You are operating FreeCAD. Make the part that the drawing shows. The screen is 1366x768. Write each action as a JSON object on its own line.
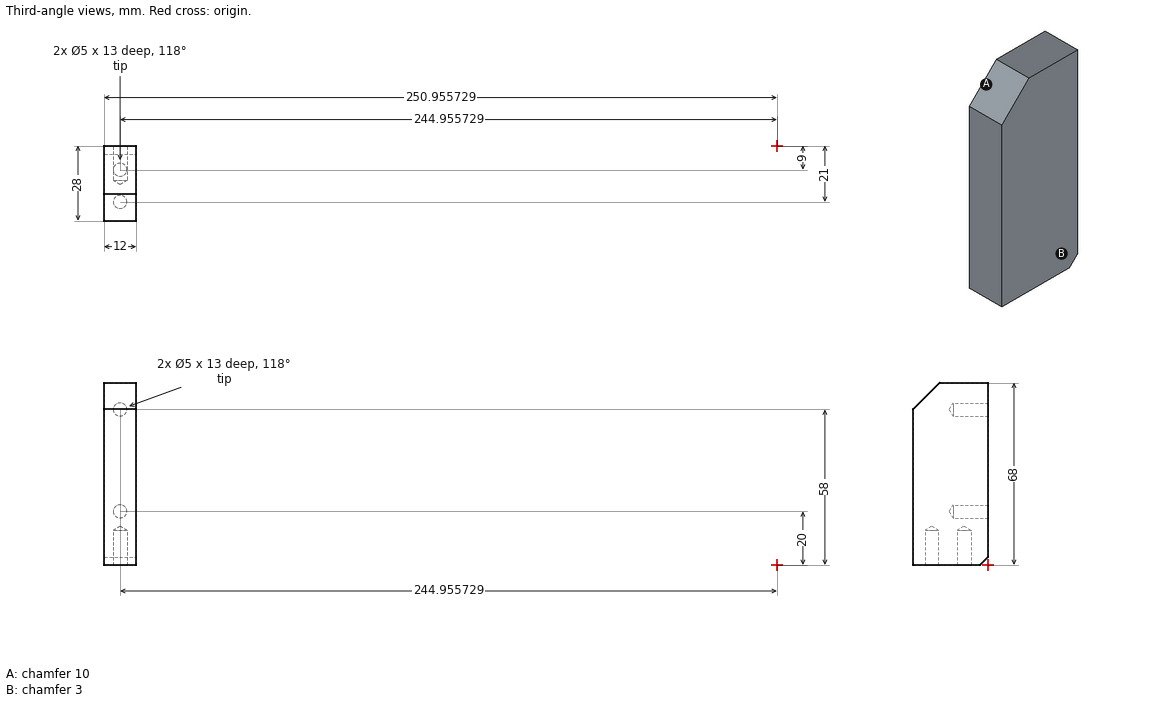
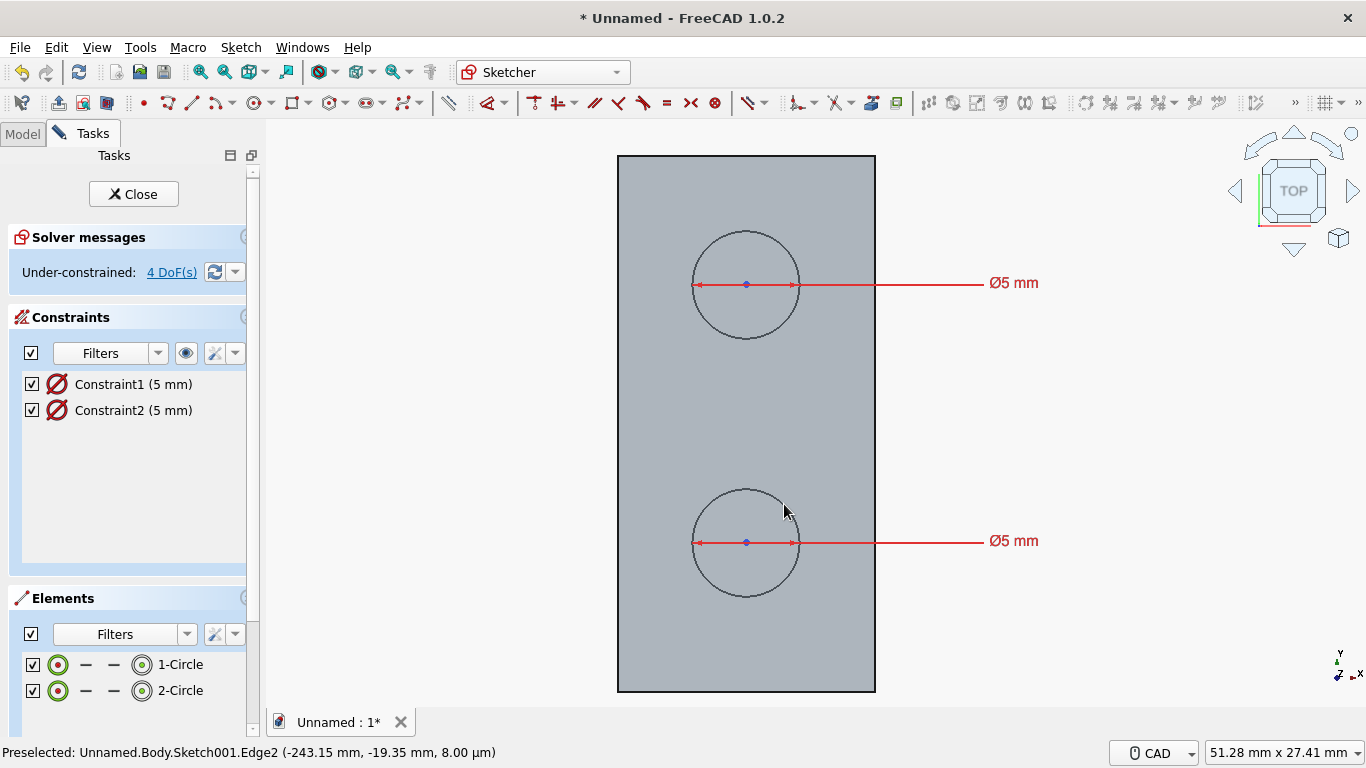
{"action": "left_click", "coordinate": [488, 104]}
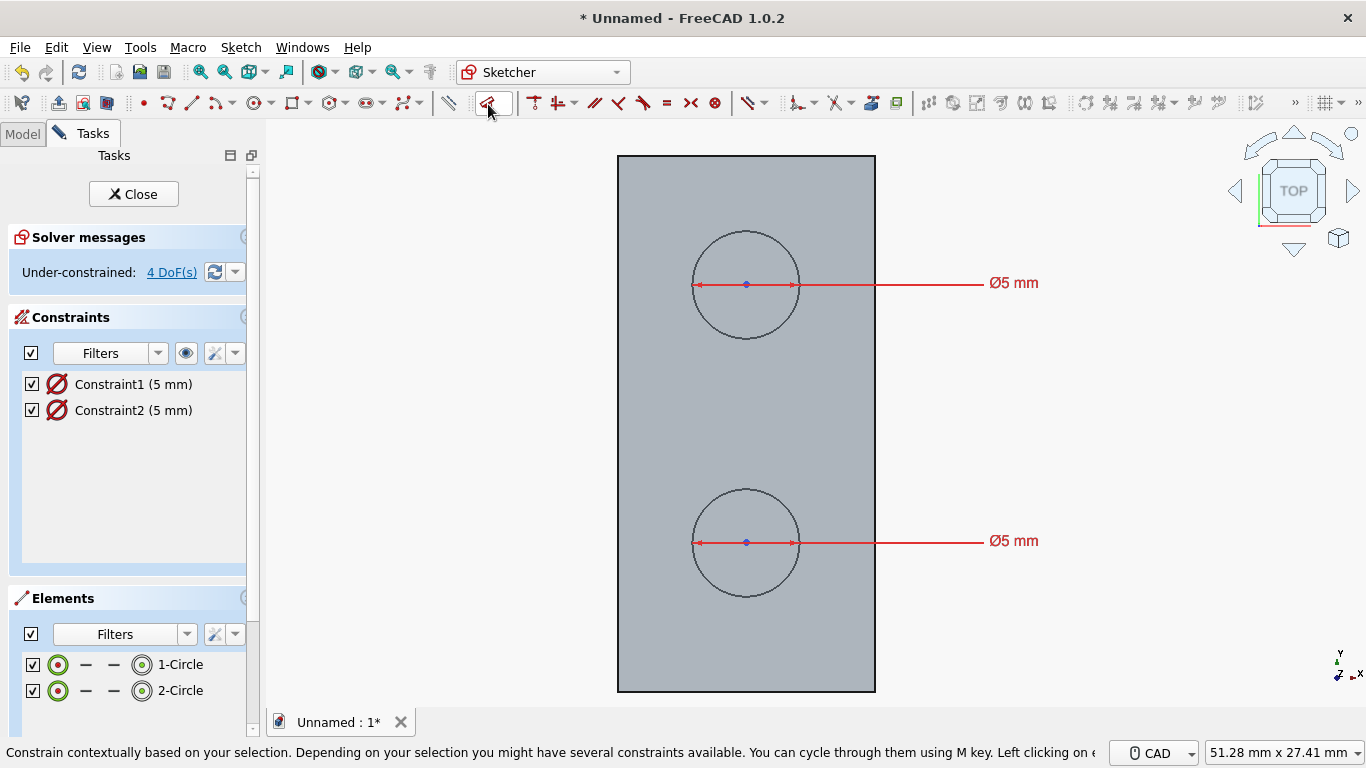
{"action": "left_click", "coordinate": [746, 285]}
{"action": "left_click", "coordinate": [712, 216]}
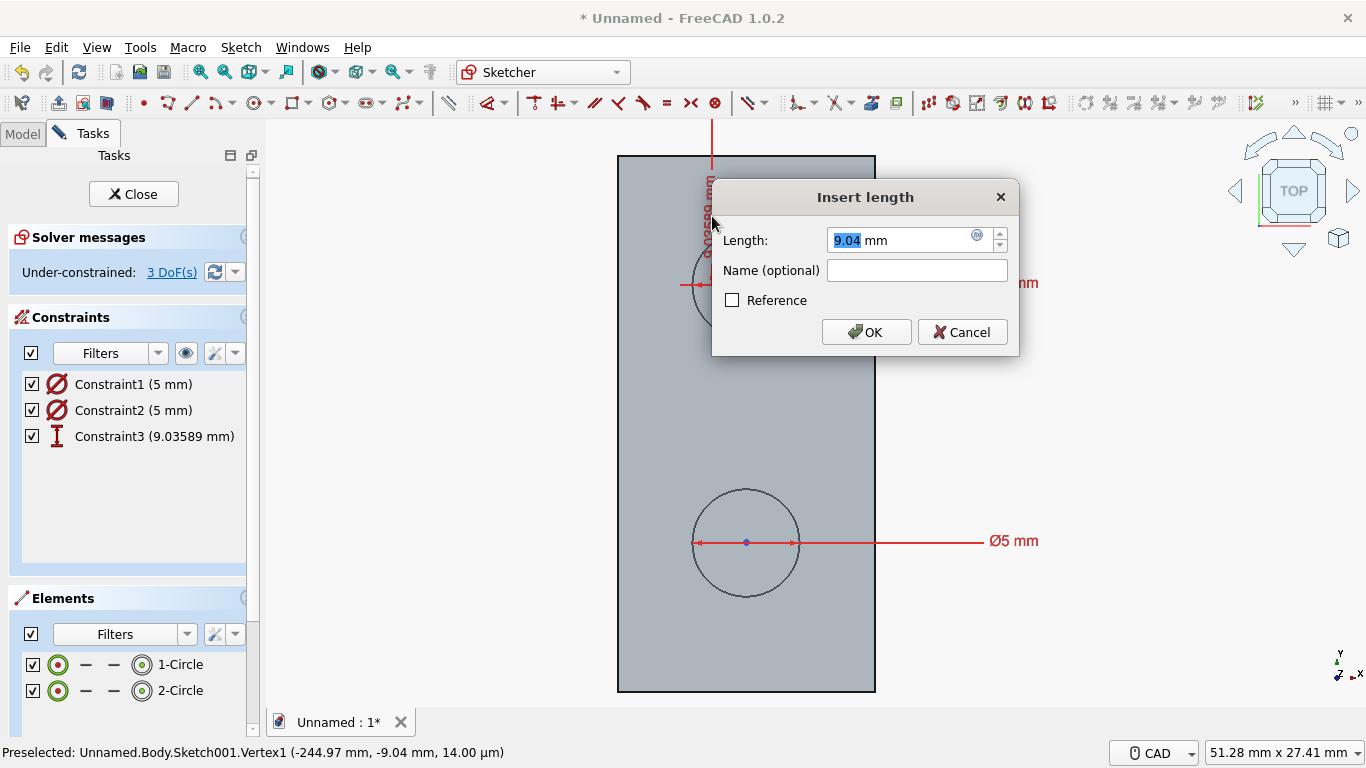
{"action": "type", "text": "9"}
{"action": "key", "text": "Return"}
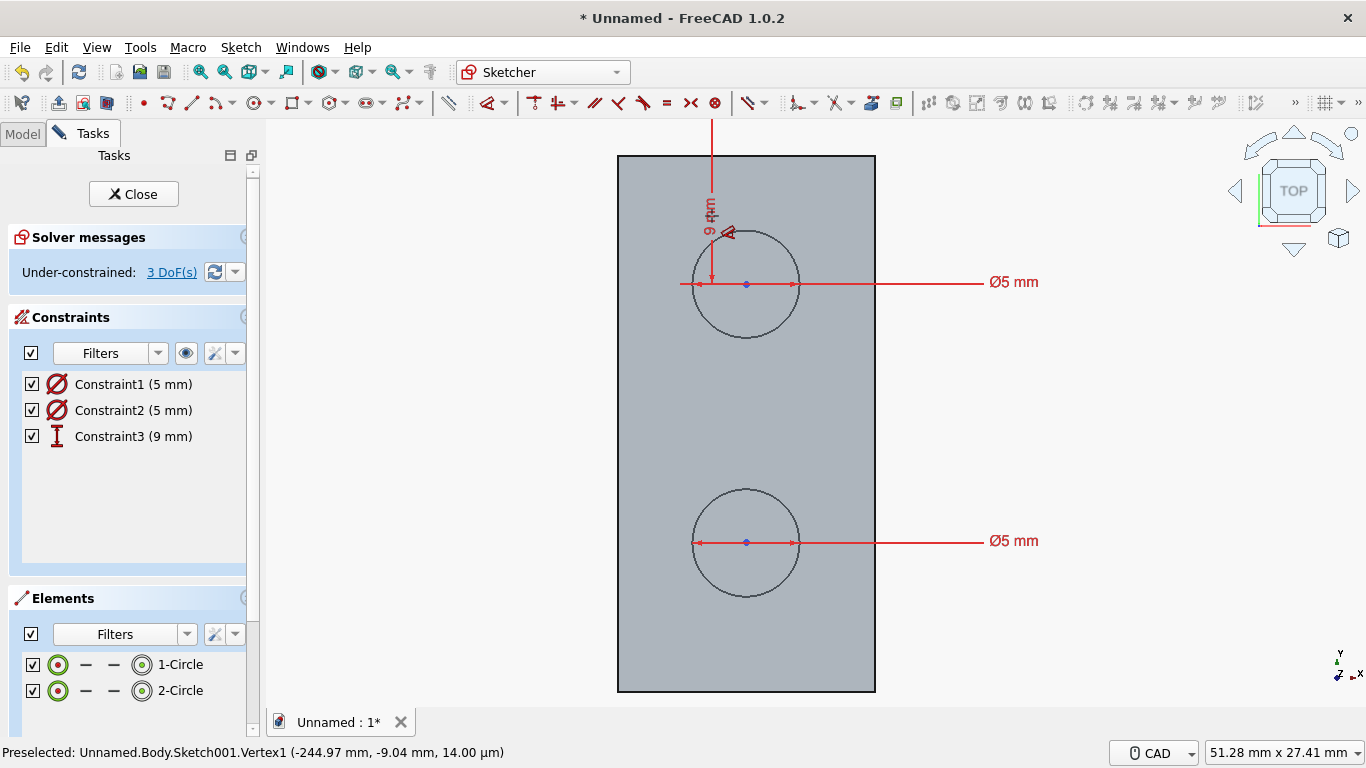
{"action": "left_click", "coordinate": [746, 543]}
{"action": "left_click", "coordinate": [712, 345]}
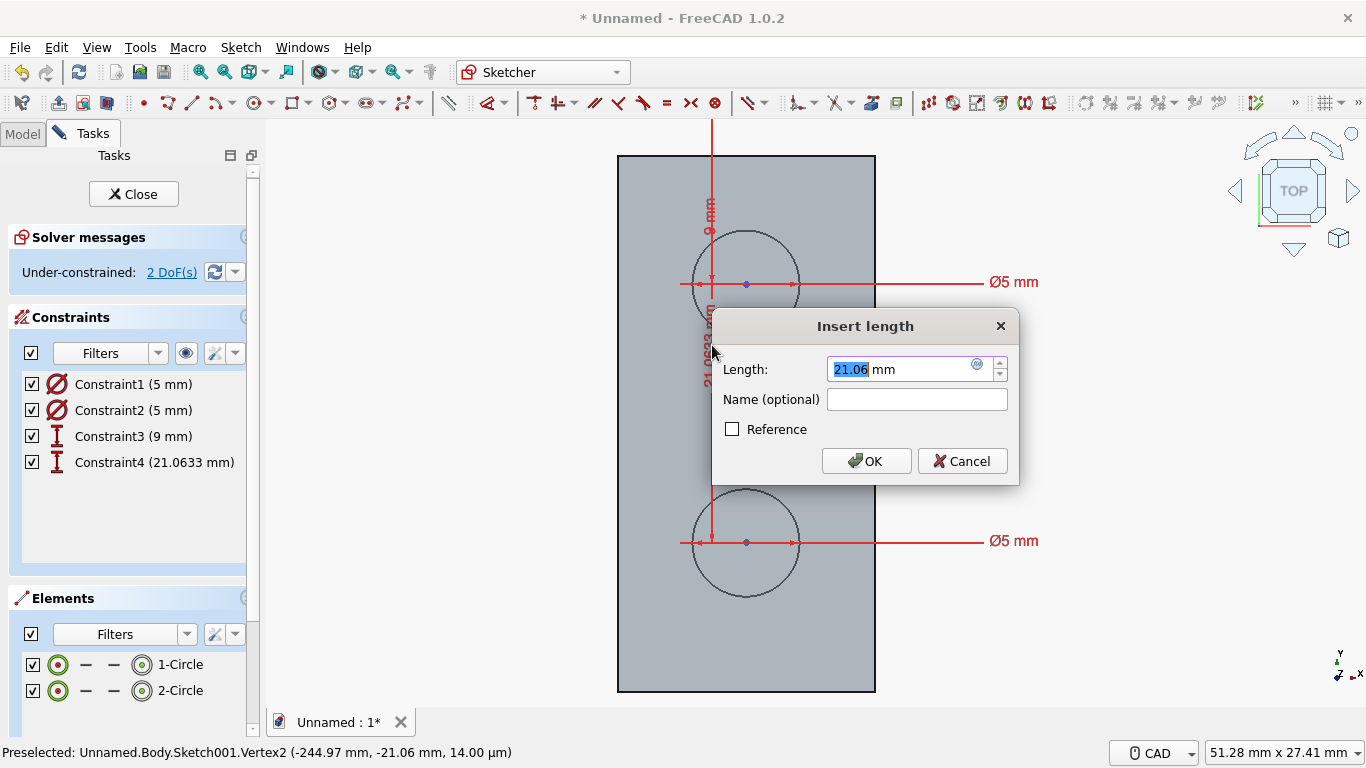
{"action": "type", "text": "21"}
{"action": "key", "text": "Return"}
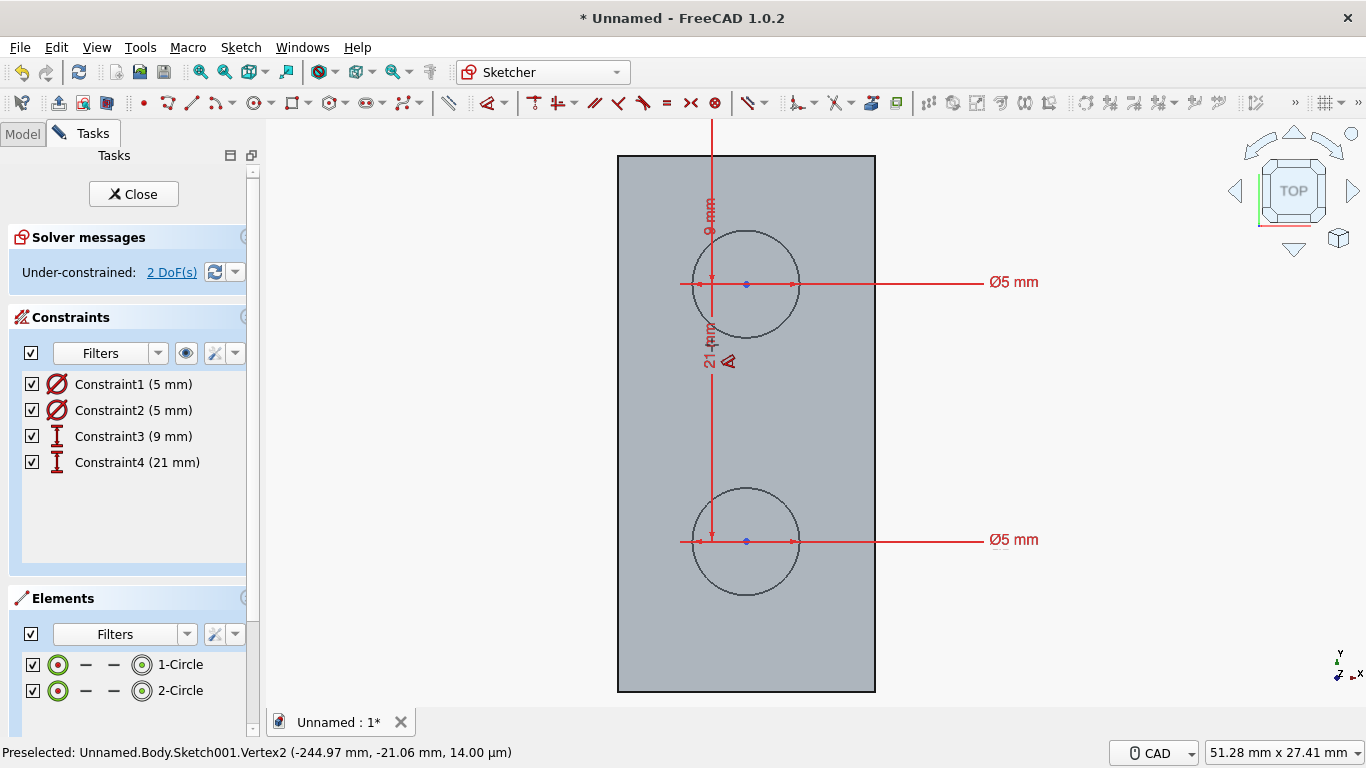
{"action": "left_click", "coordinate": [746, 284]}
{"action": "left_click", "coordinate": [973, 318]}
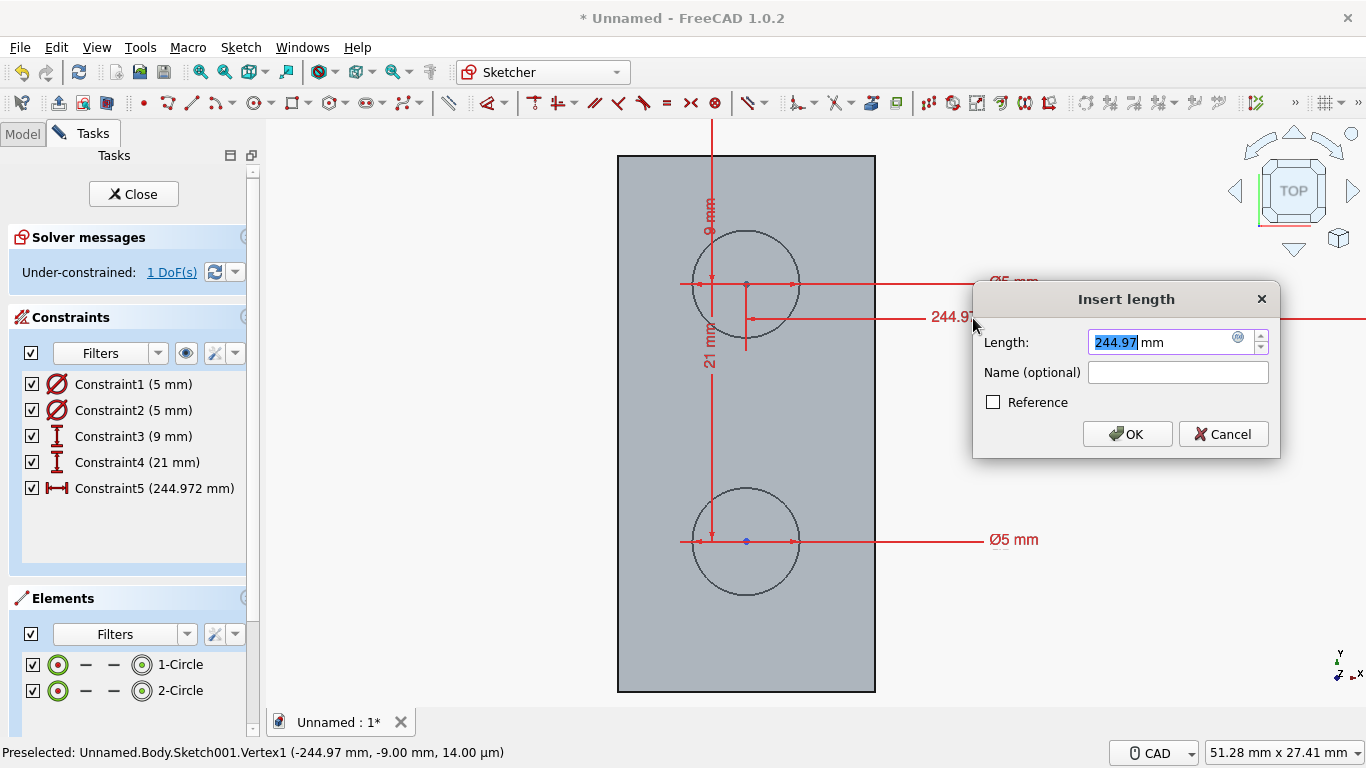
{"action": "type", "text": "244.955729"}
{"action": "key", "text": "Return"}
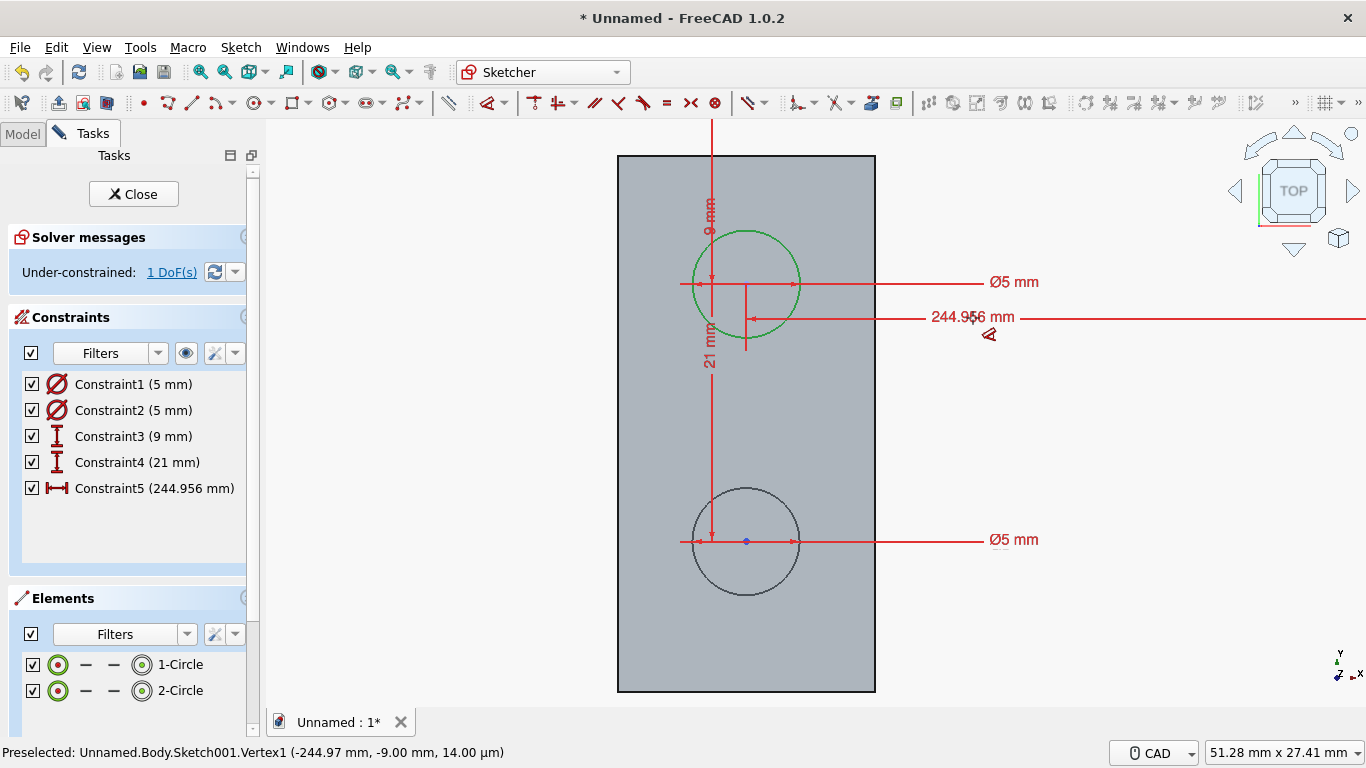
{"action": "left_click", "coordinate": [746, 542]}
{"action": "left_click", "coordinate": [973, 576]}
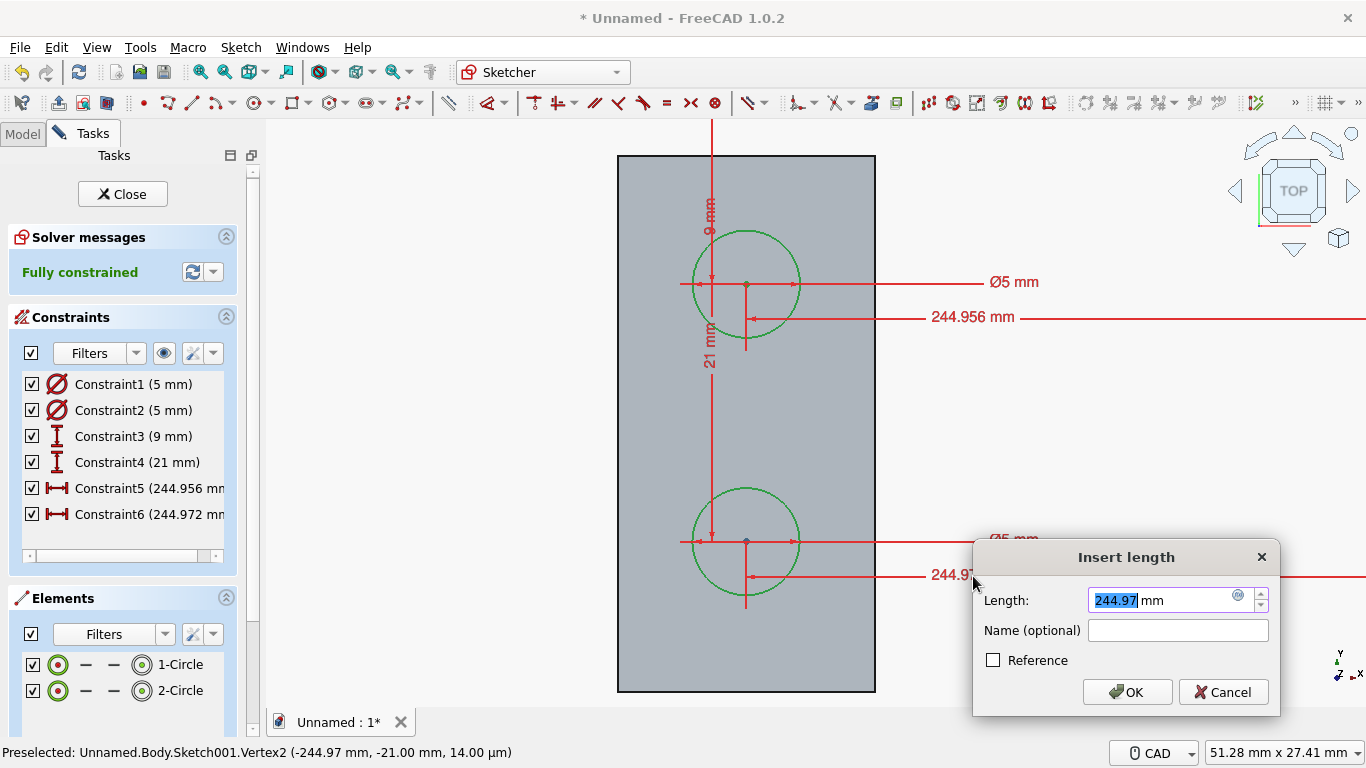
{"action": "type", "text": "244.955729"}
{"action": "key", "text": "Return"}
{"action": "key", "text": "Escape"}